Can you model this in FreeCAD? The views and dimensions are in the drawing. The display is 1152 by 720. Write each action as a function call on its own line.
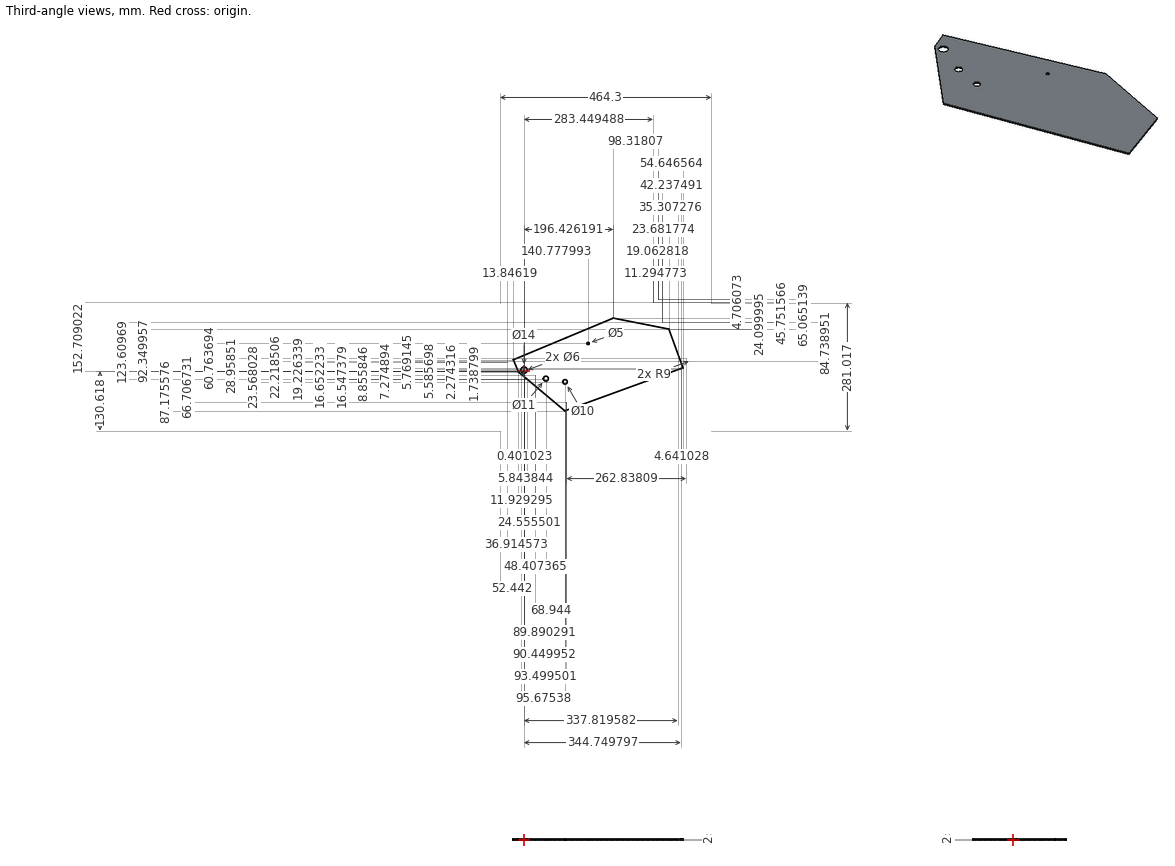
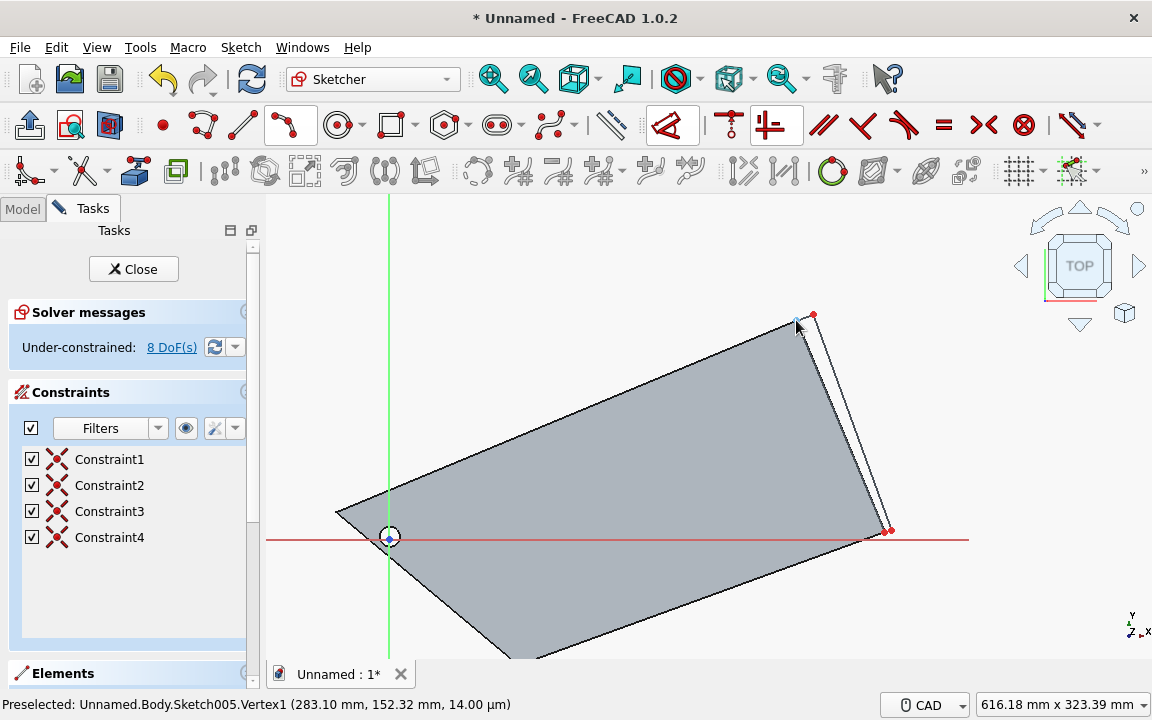
scroll(892, 530, up, 7)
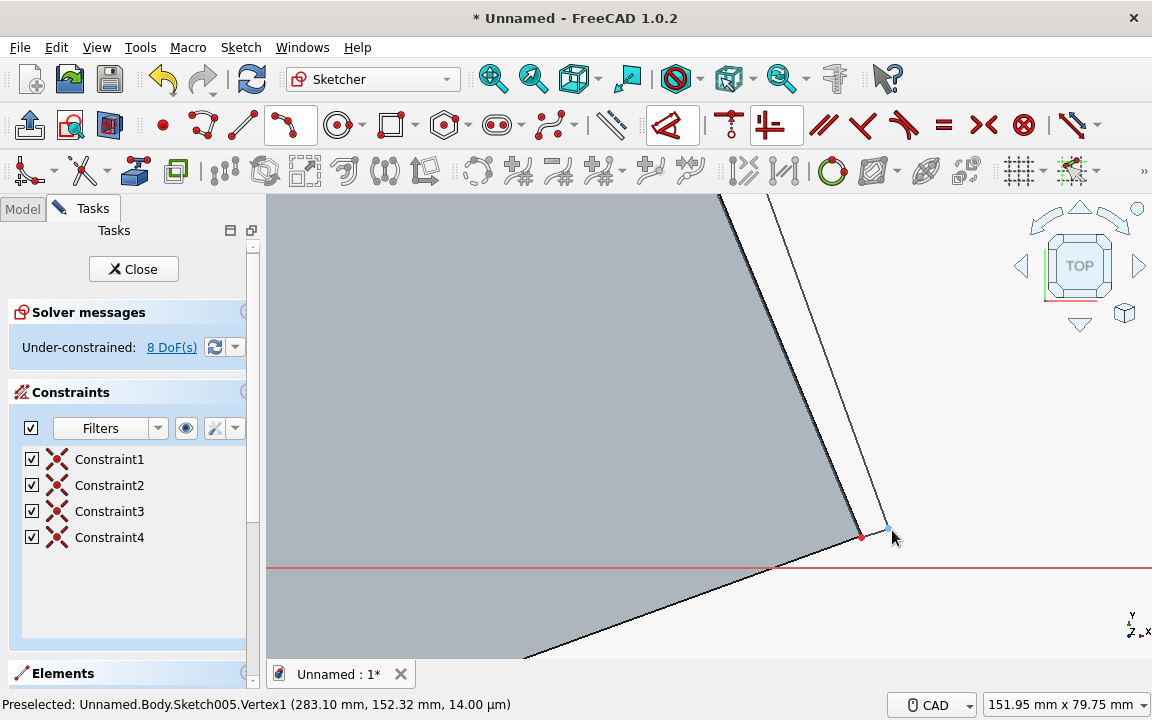
click(889, 529)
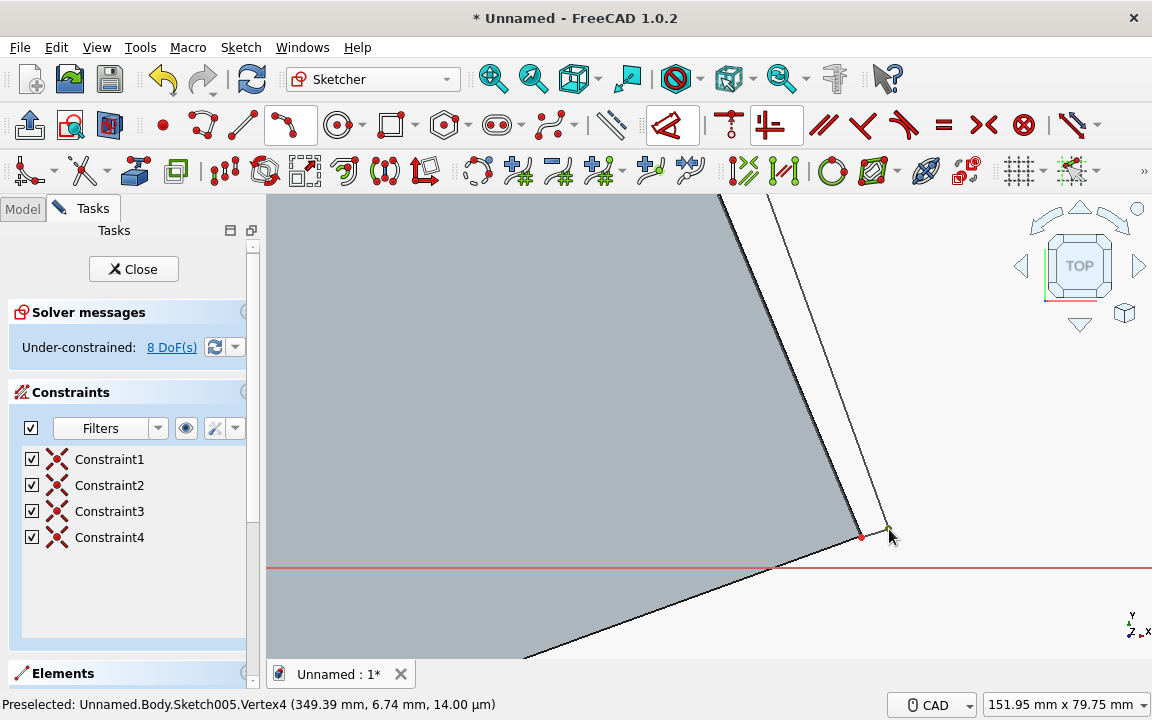
key(i)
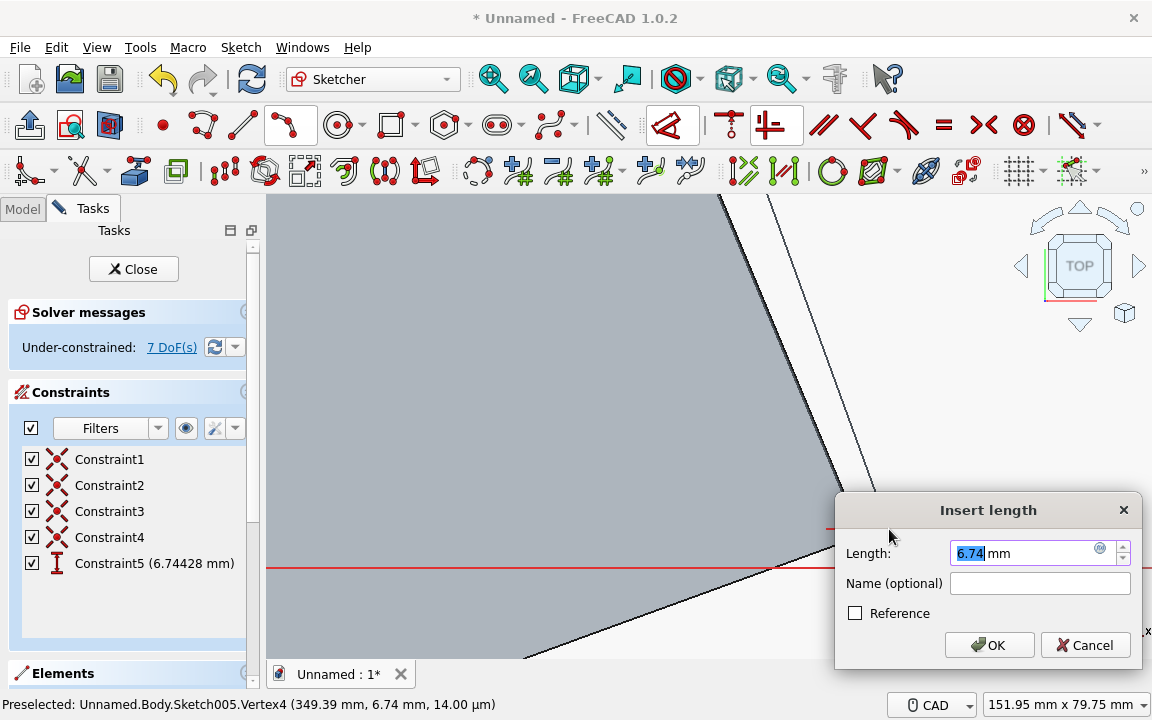
text(7.274894)
key(Return)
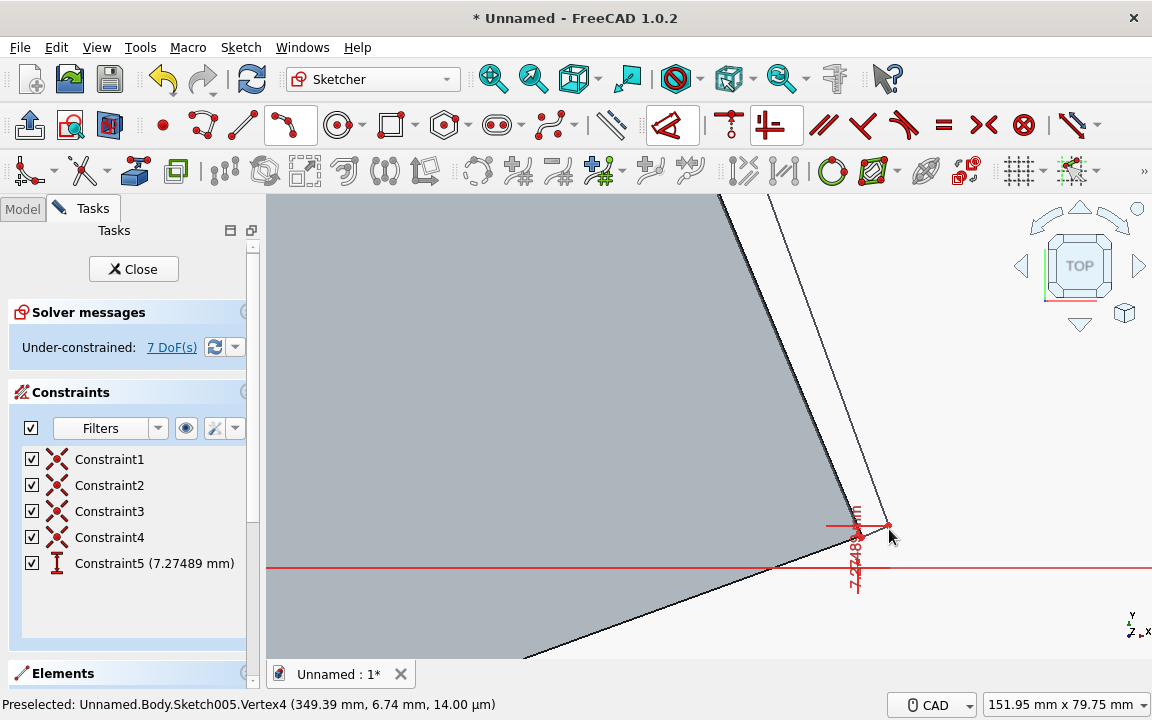
click(861, 538)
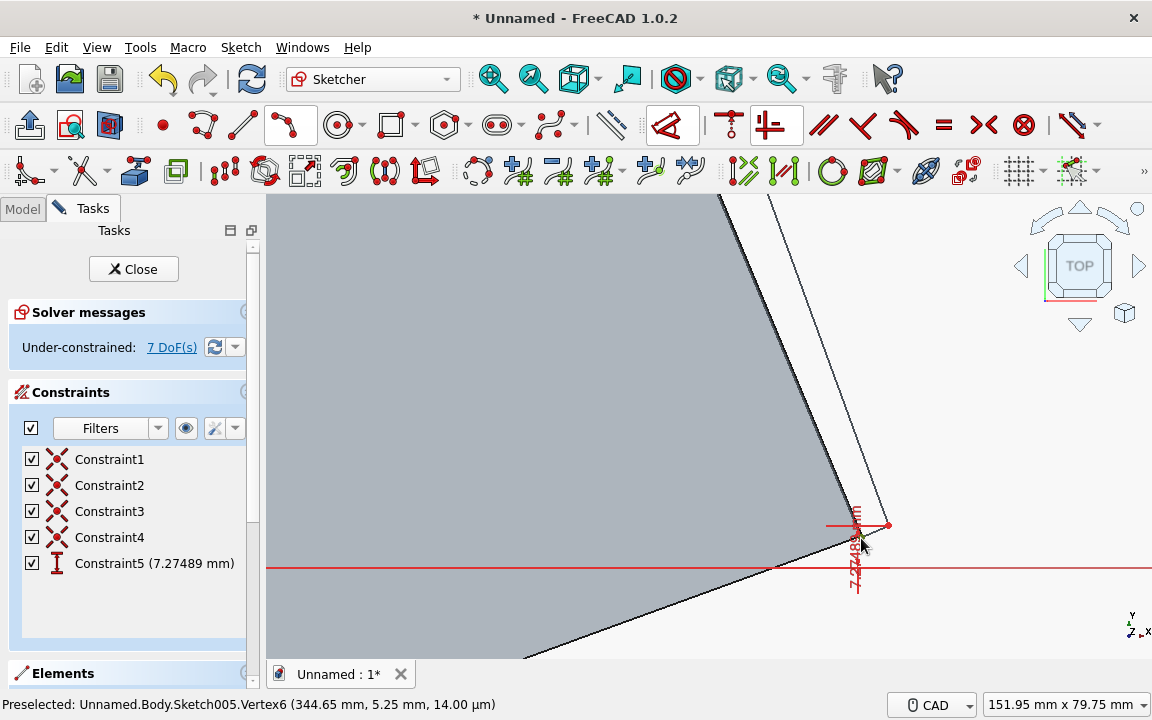
key(i)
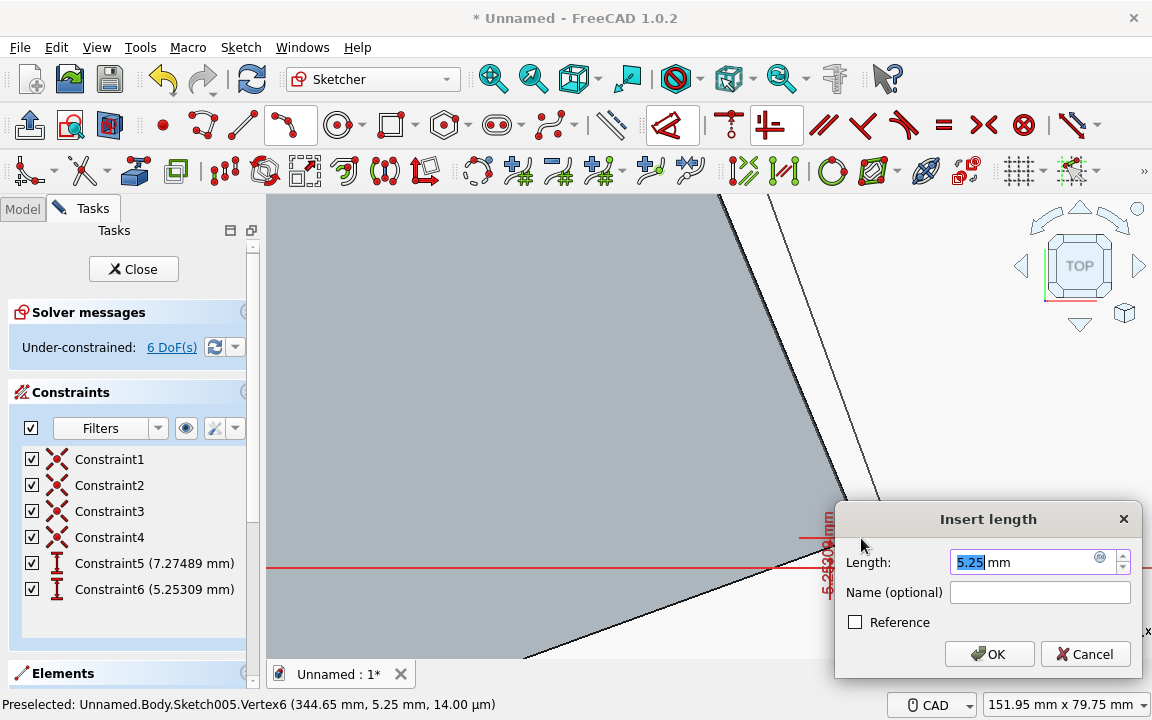
text(5.585698)
key(Return)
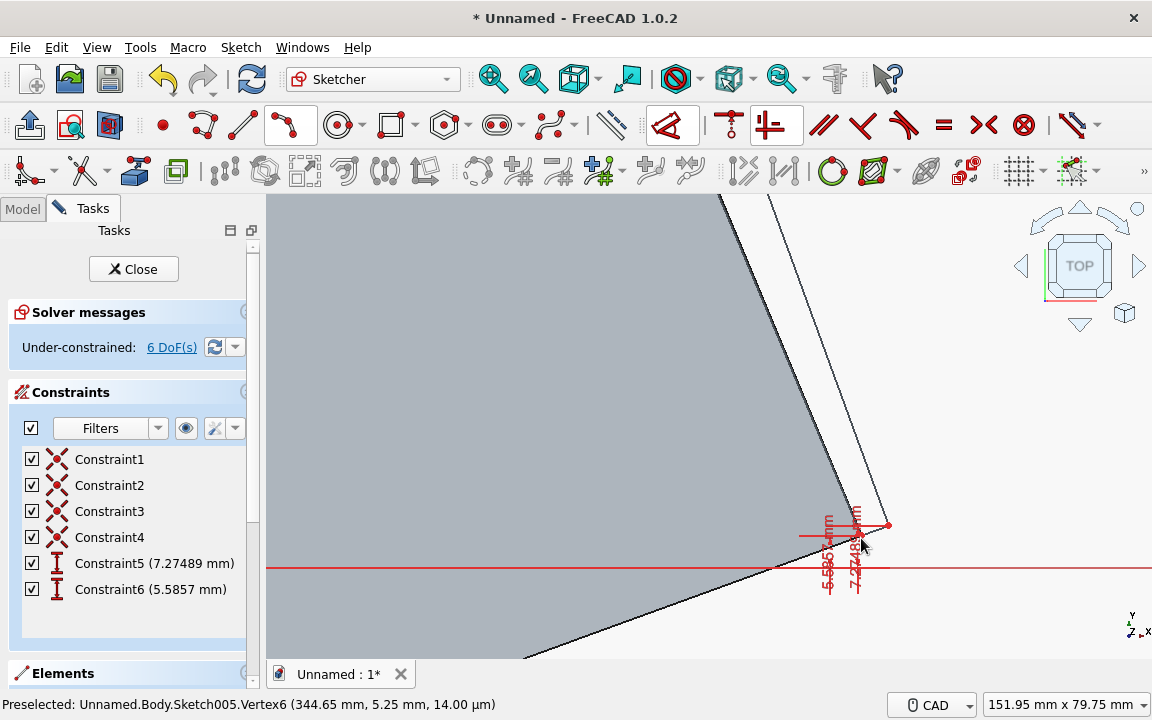
scroll(893, 530, down, 7)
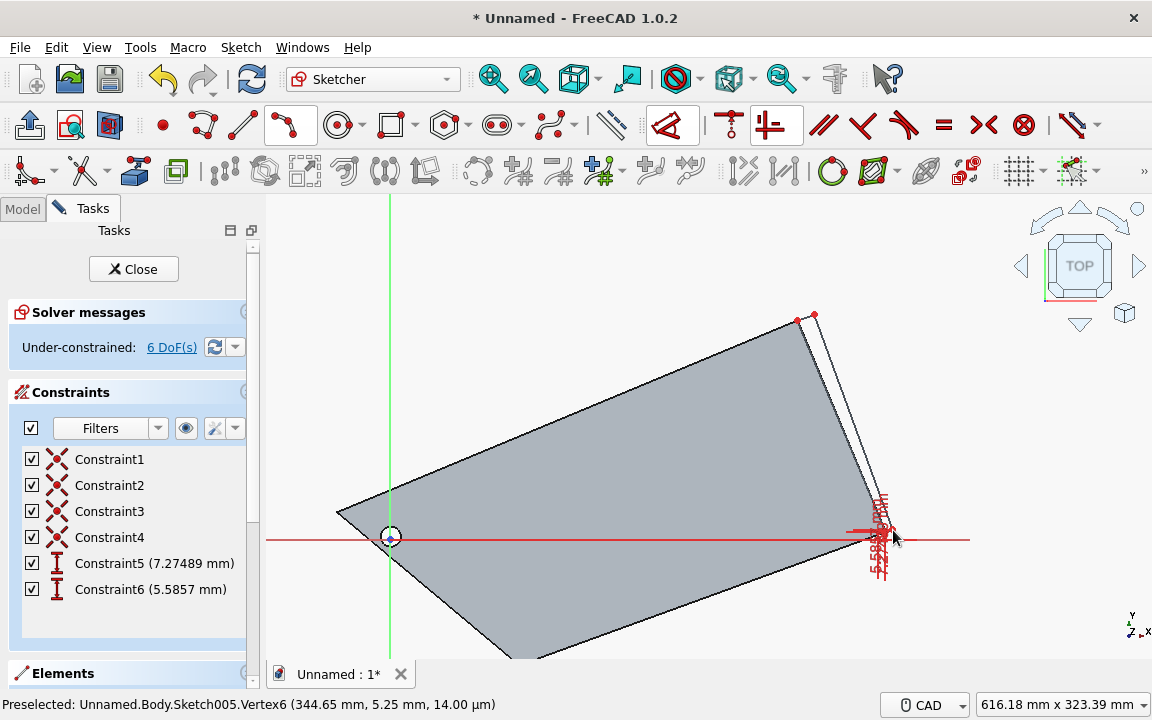
scroll(802, 319, up, 9)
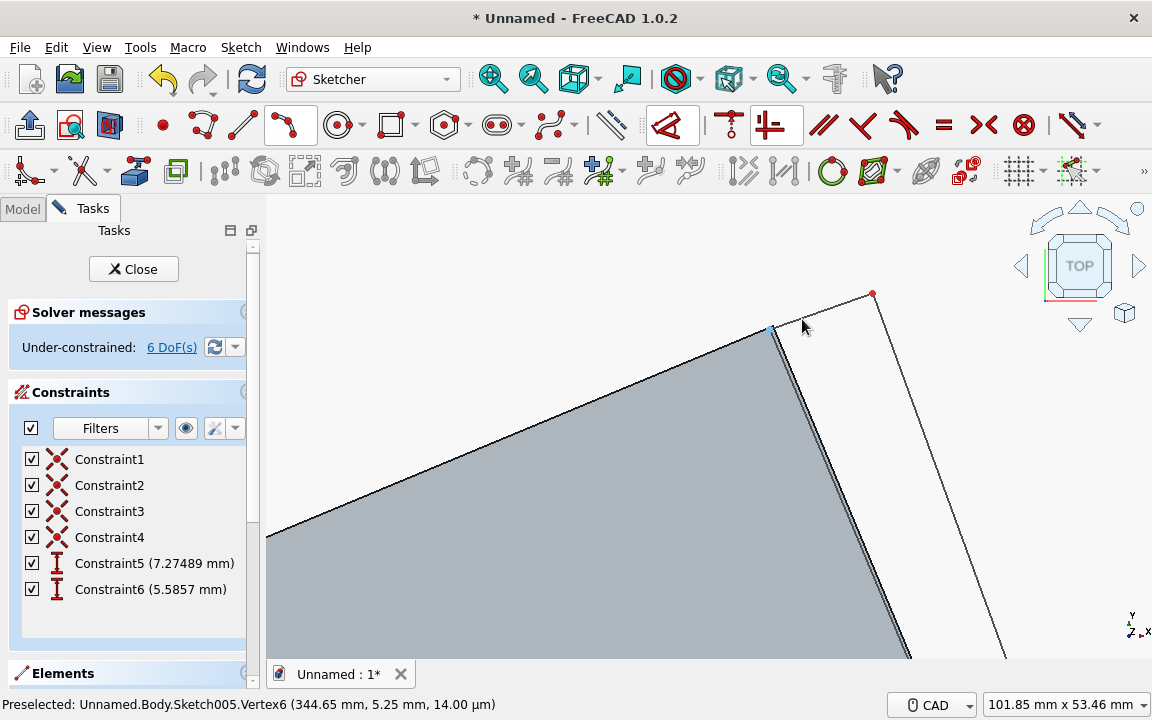
click(801, 319)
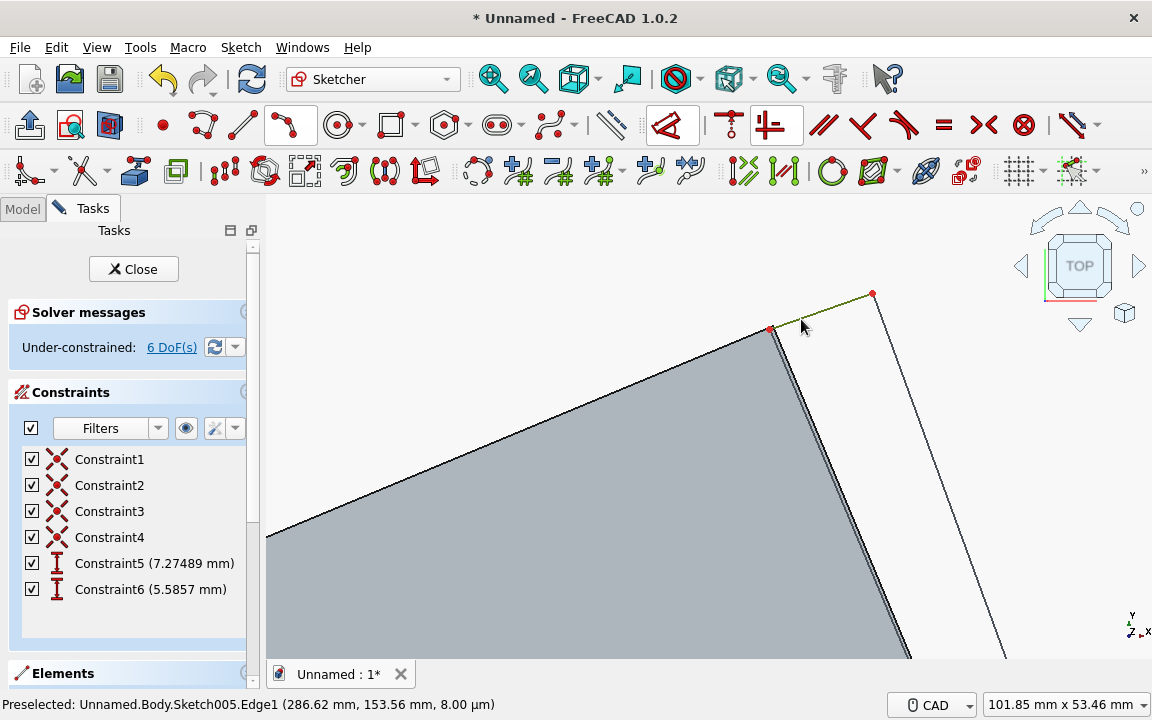
key(i)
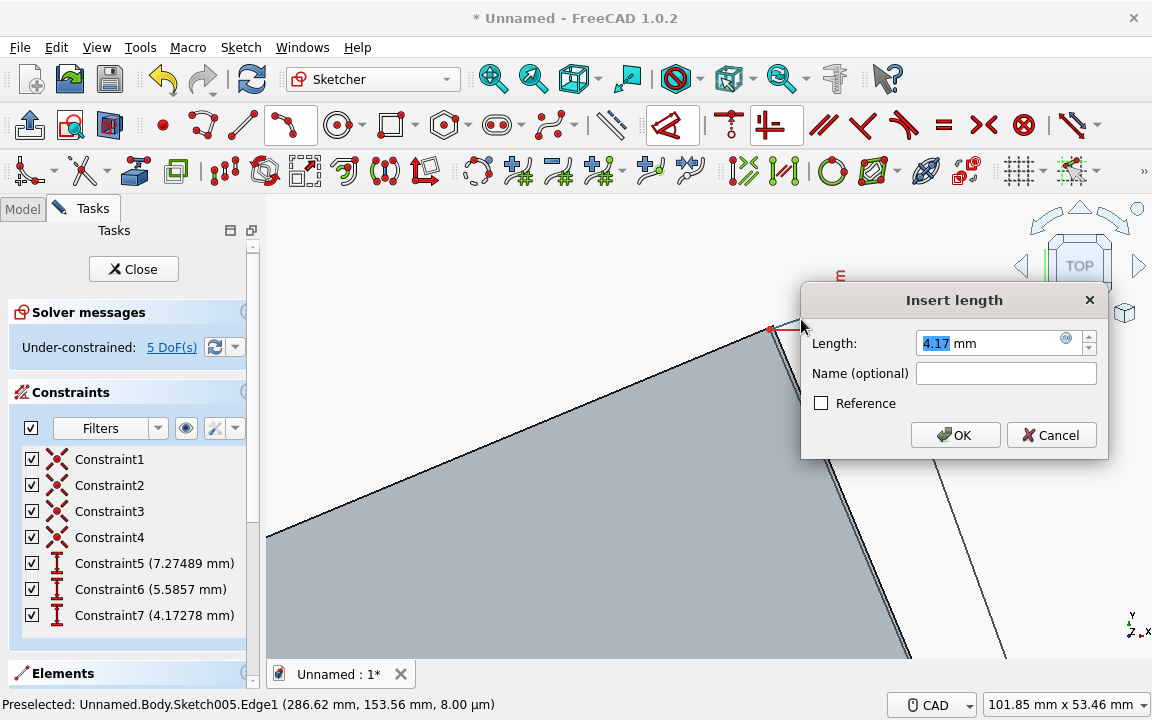
text(4.706073)
key(Return)